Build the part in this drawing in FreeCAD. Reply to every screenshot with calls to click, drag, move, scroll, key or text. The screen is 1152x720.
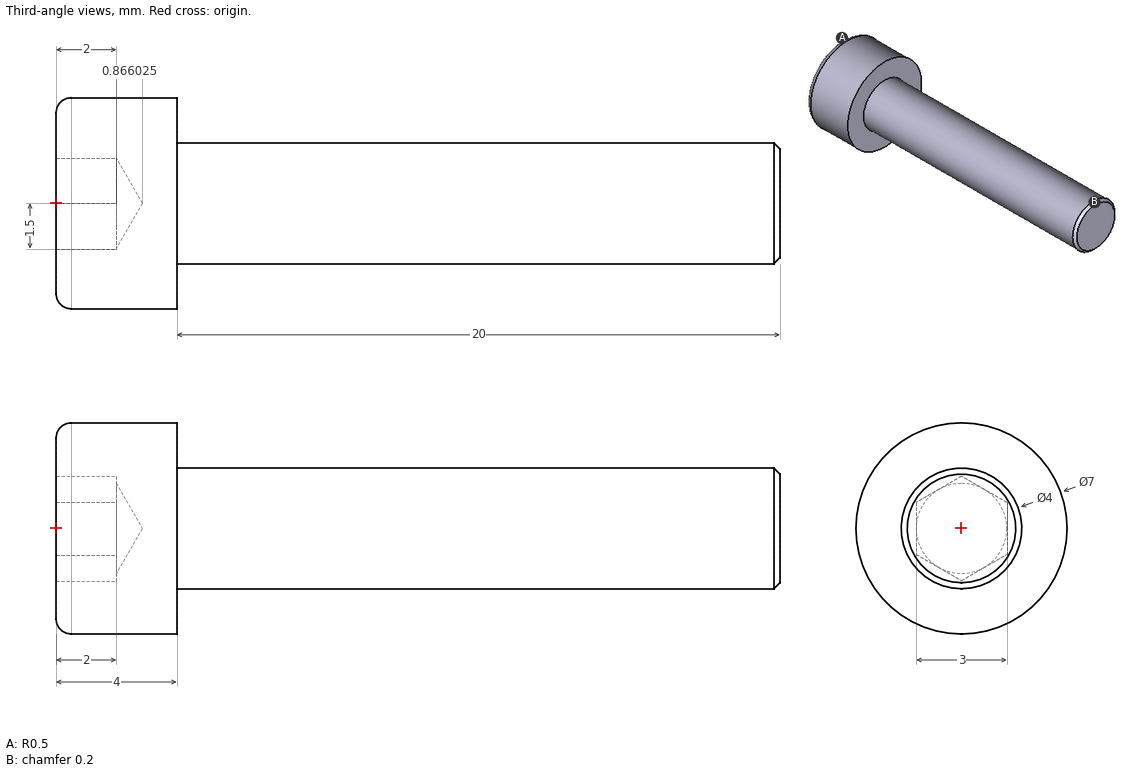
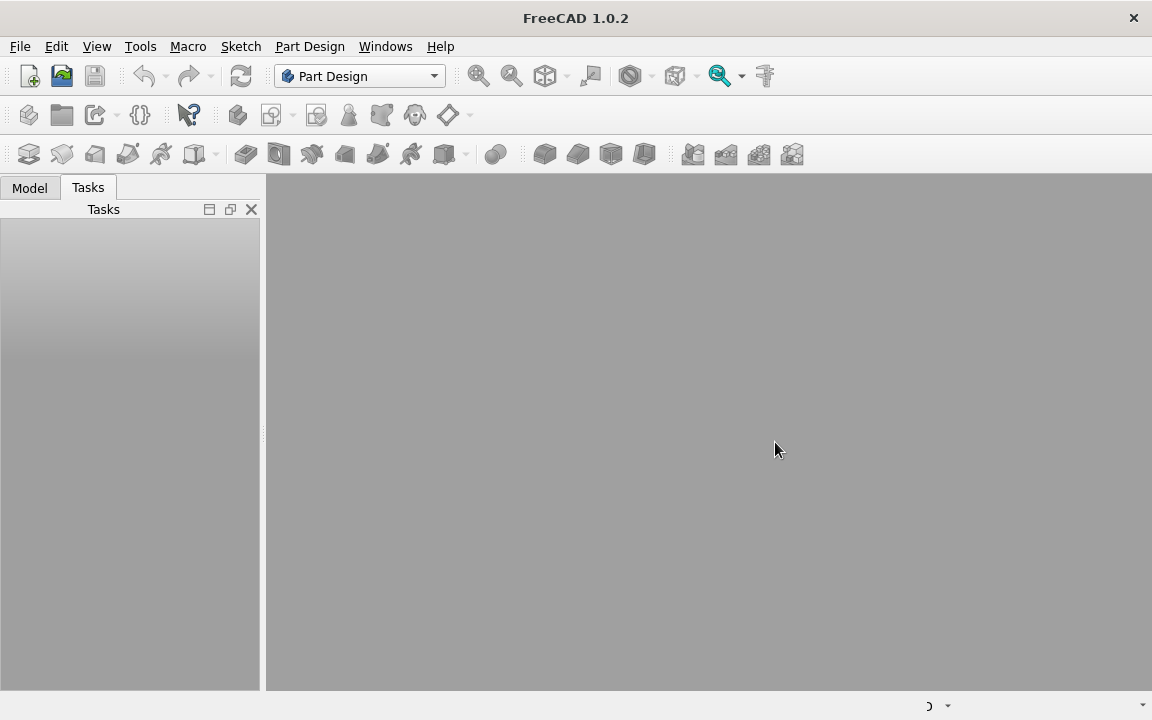
click(29, 76)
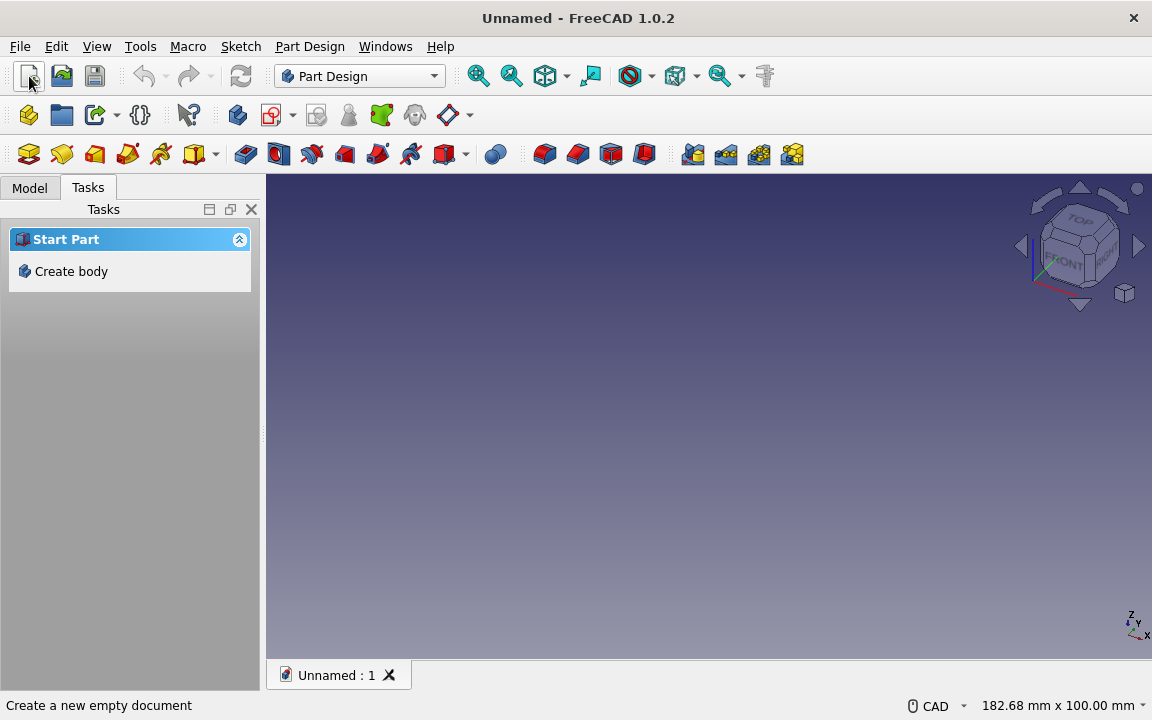
click(270, 116)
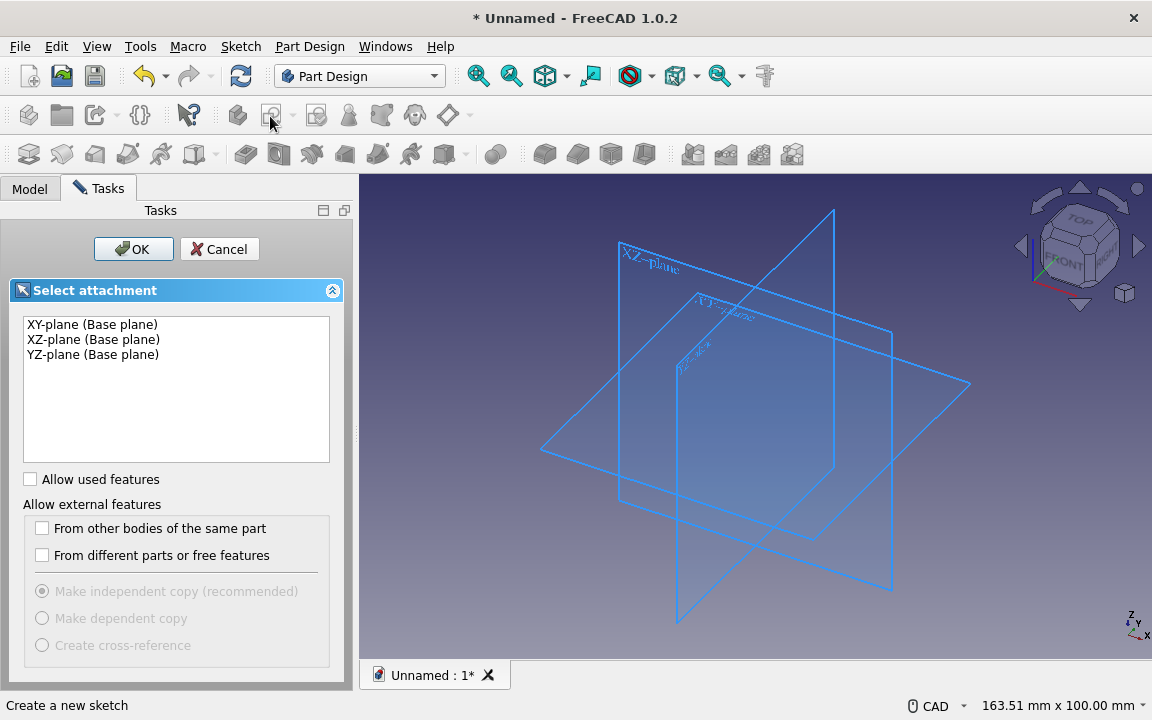
click(84, 354)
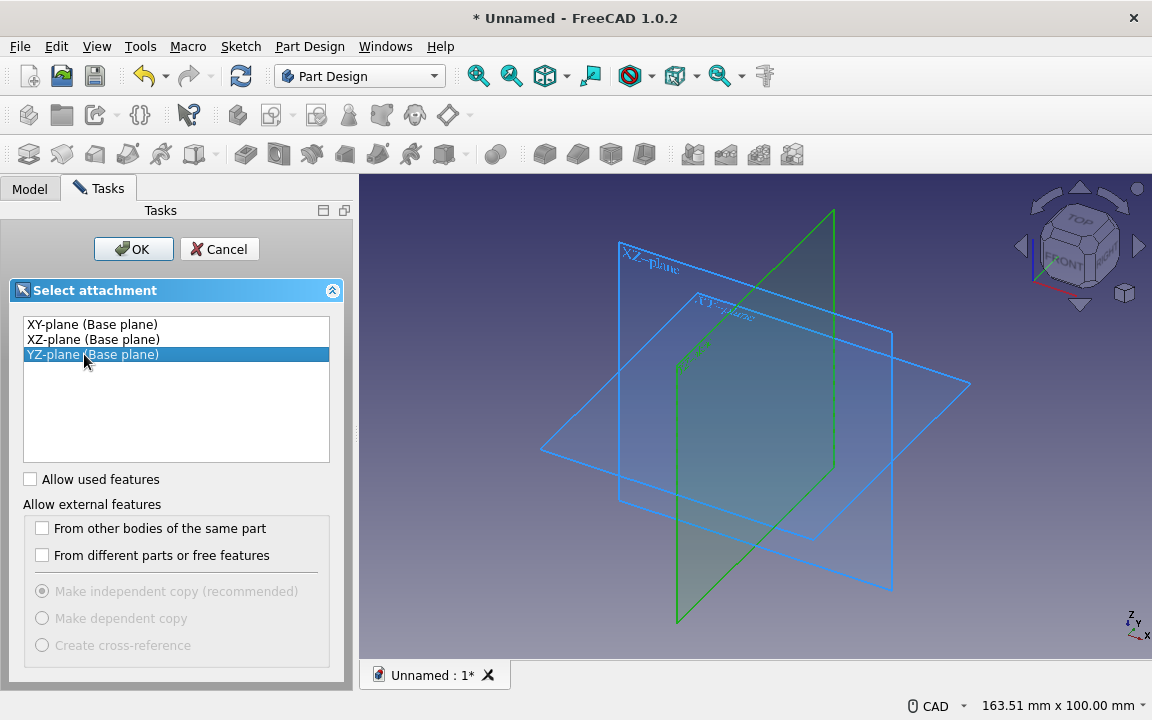
click(134, 249)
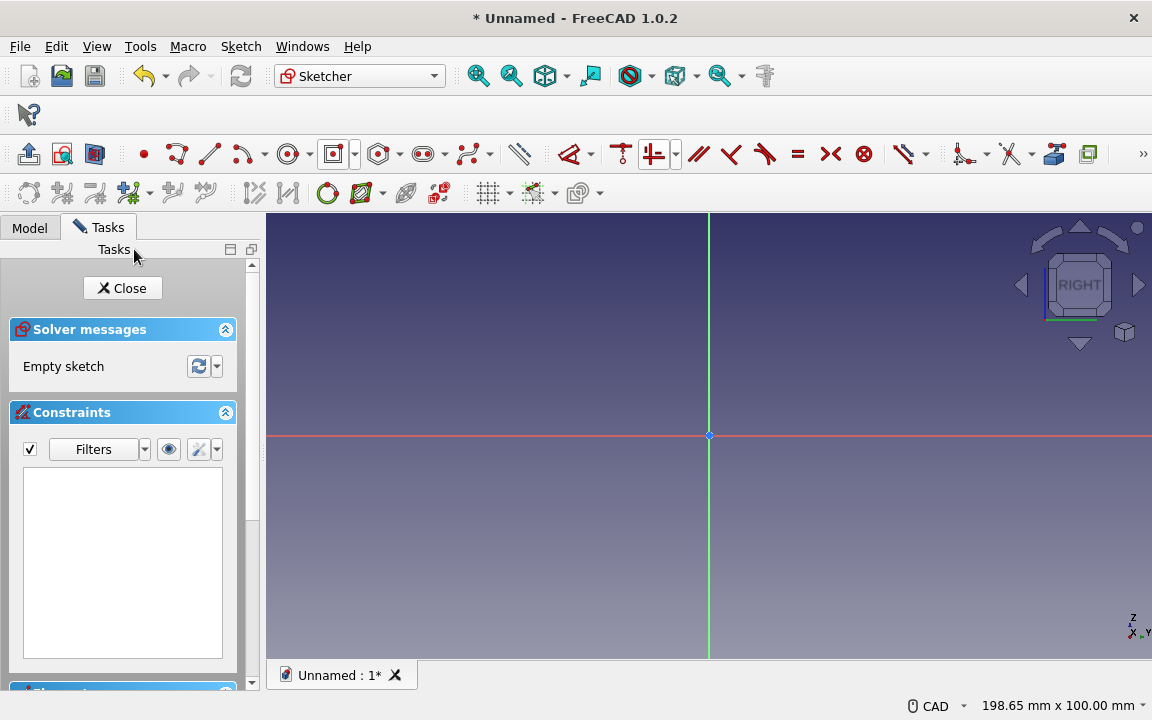
scroll(718, 436, up, 11)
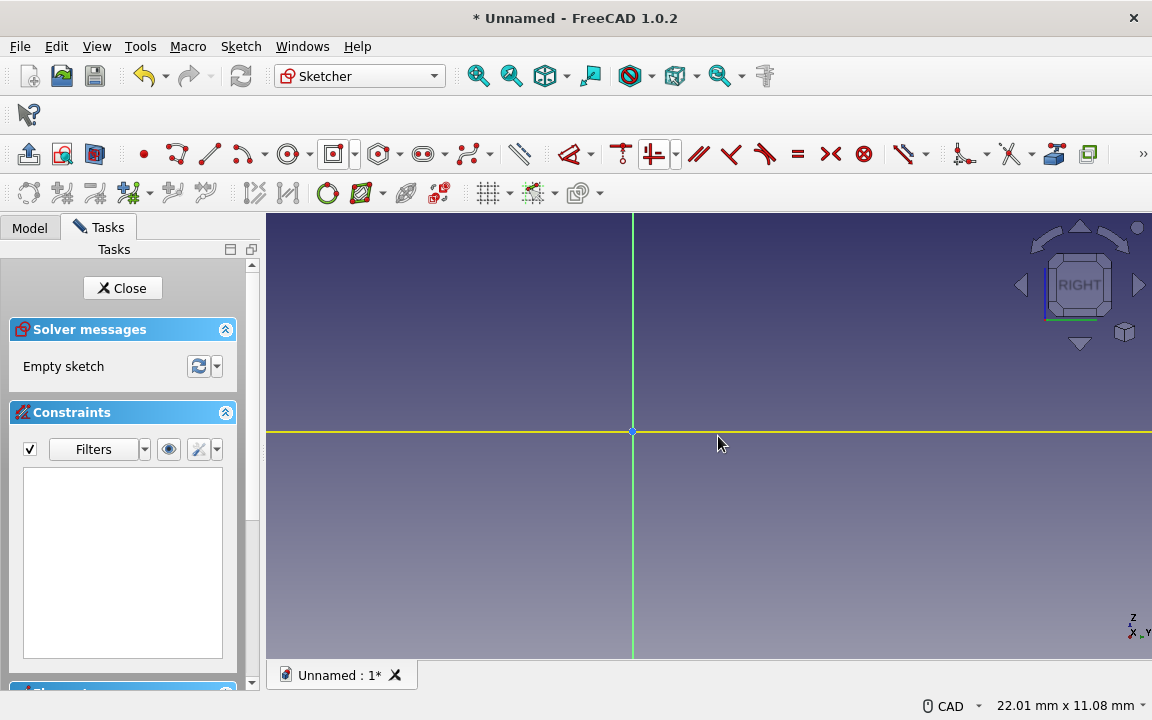
click(288, 154)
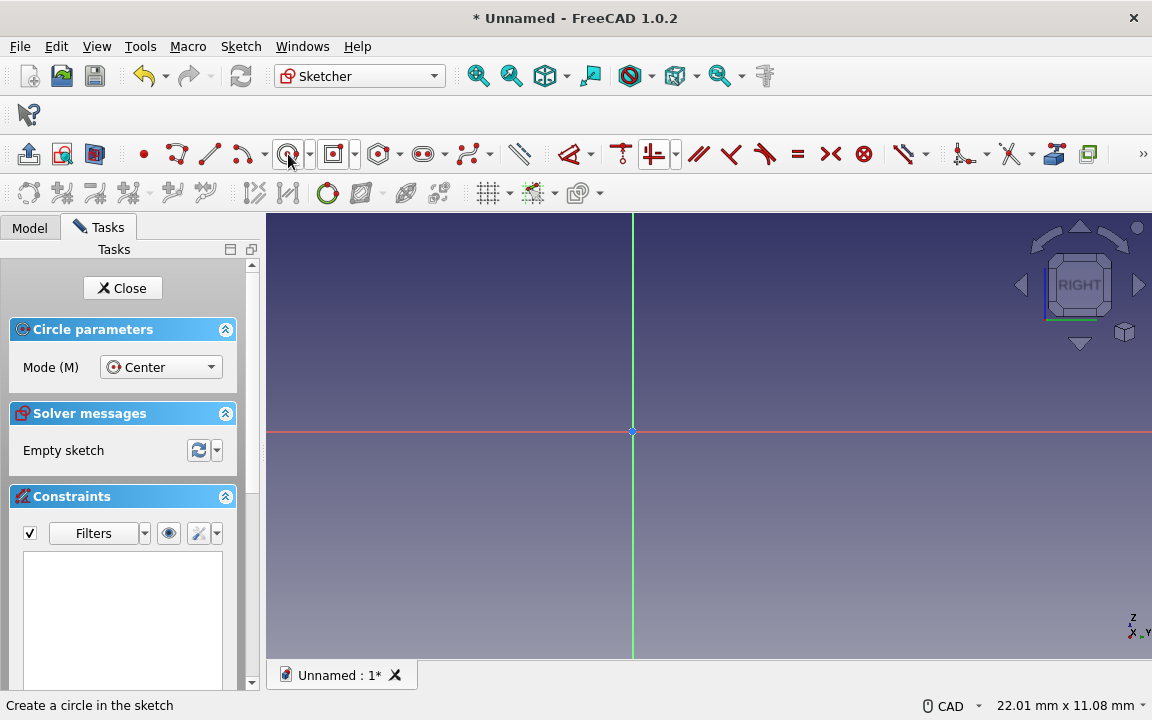
click(633, 432)
click(732, 332)
key(Escape)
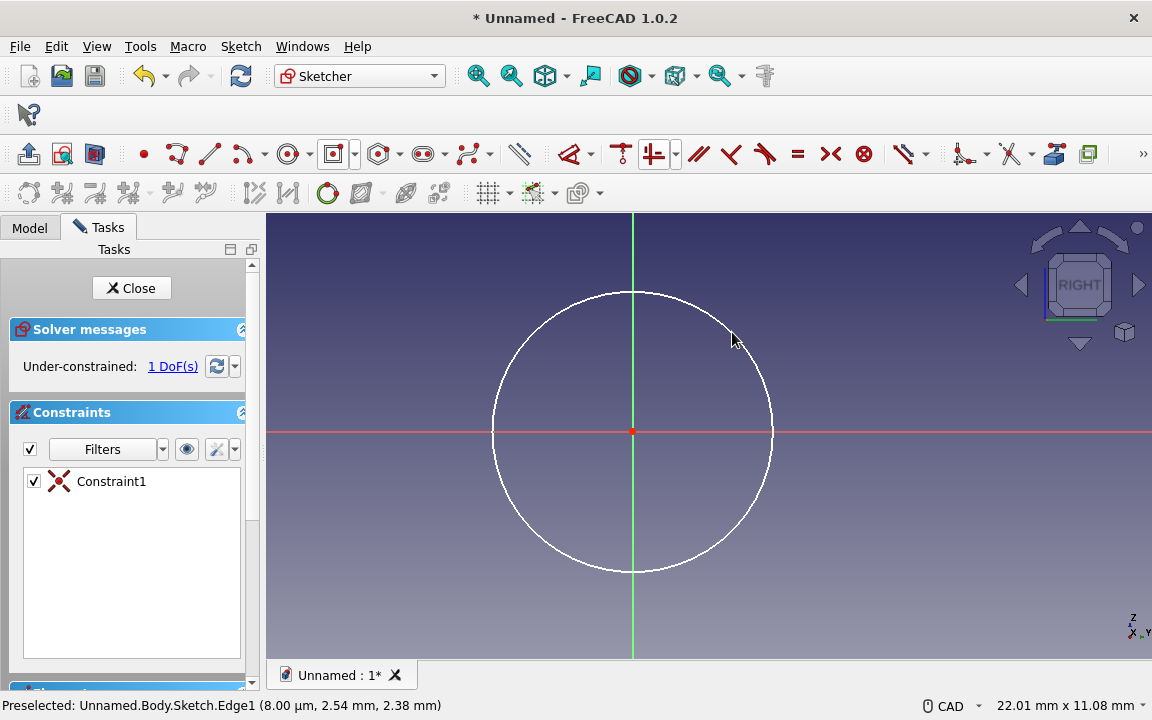
click(568, 154)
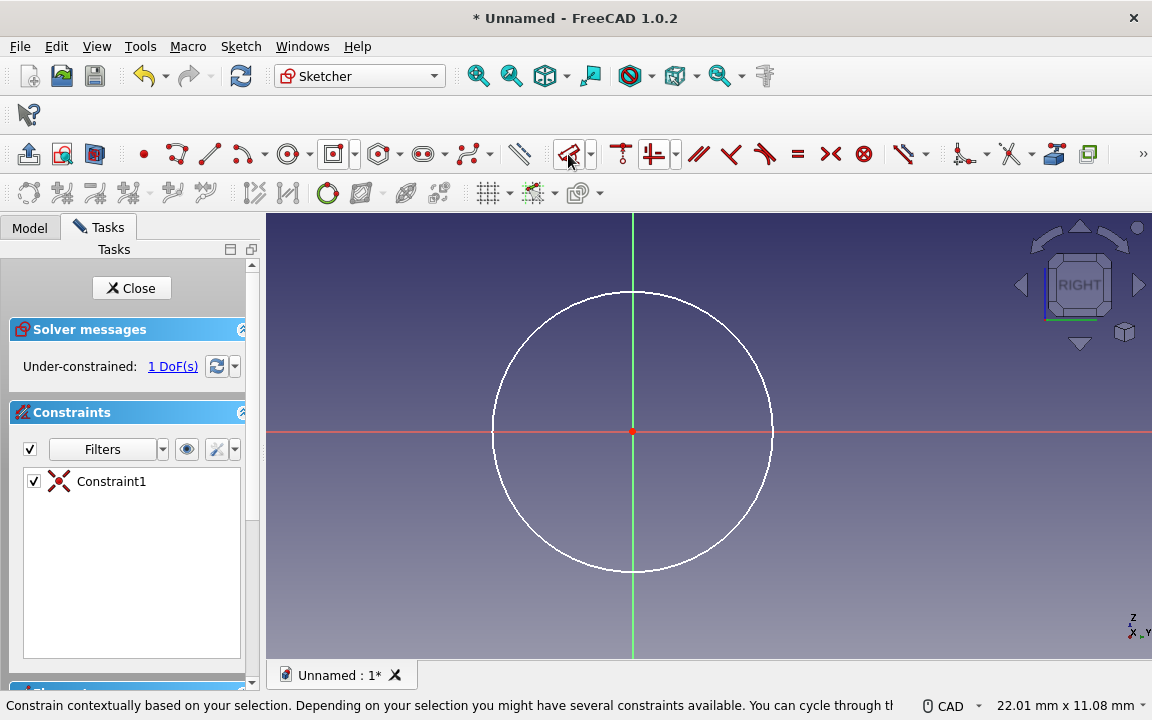
click(732, 333)
click(755, 310)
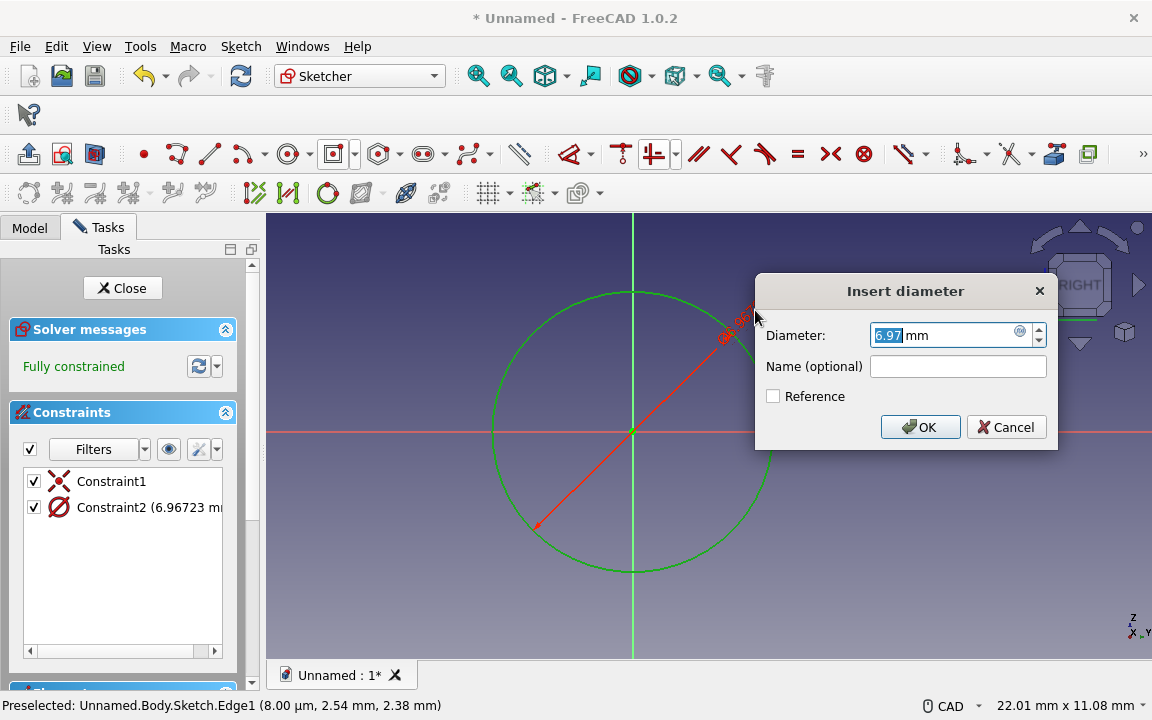
text(7)
key(Return)
key(Escape)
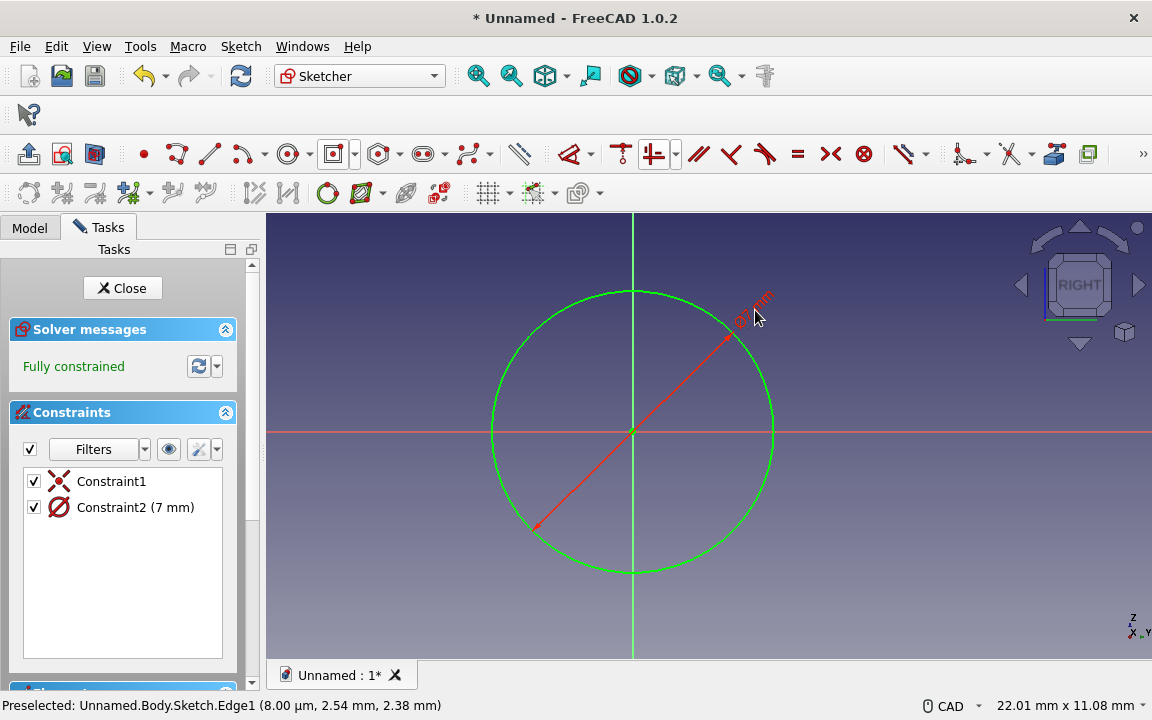
click(123, 288)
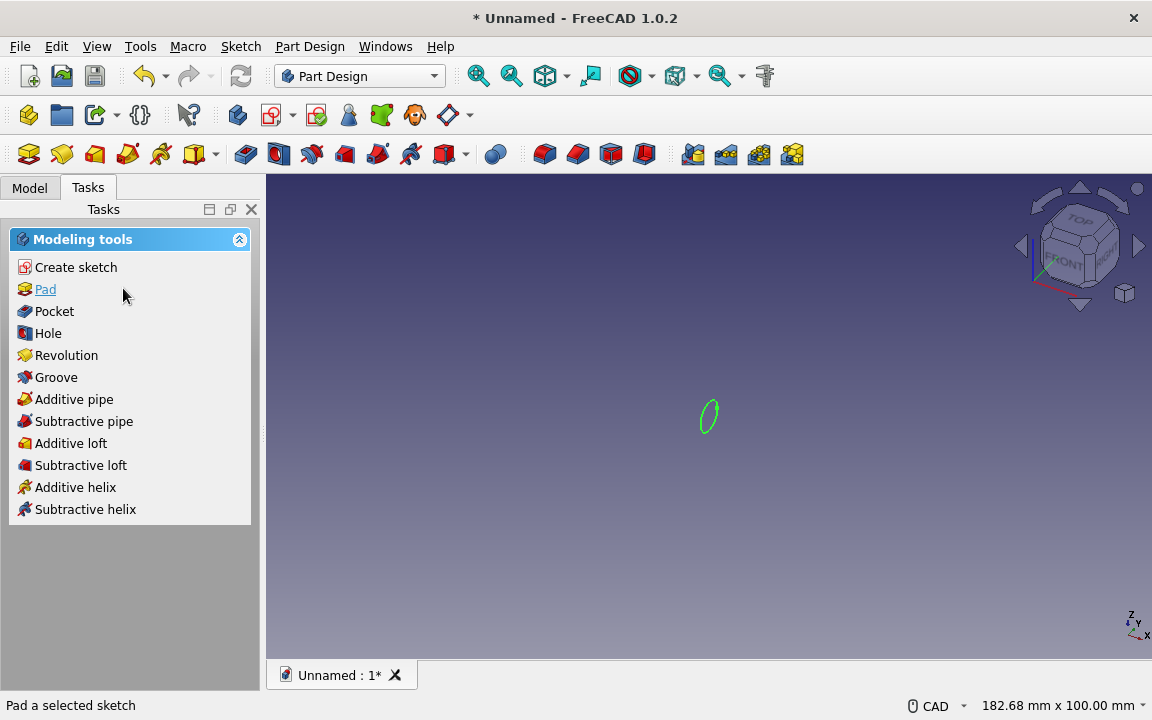
click(29, 154)